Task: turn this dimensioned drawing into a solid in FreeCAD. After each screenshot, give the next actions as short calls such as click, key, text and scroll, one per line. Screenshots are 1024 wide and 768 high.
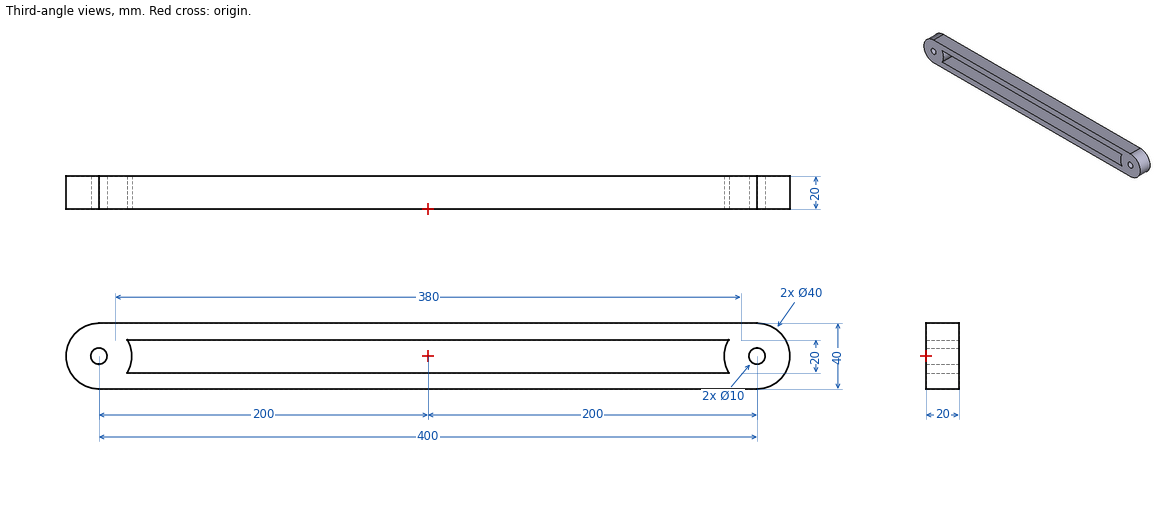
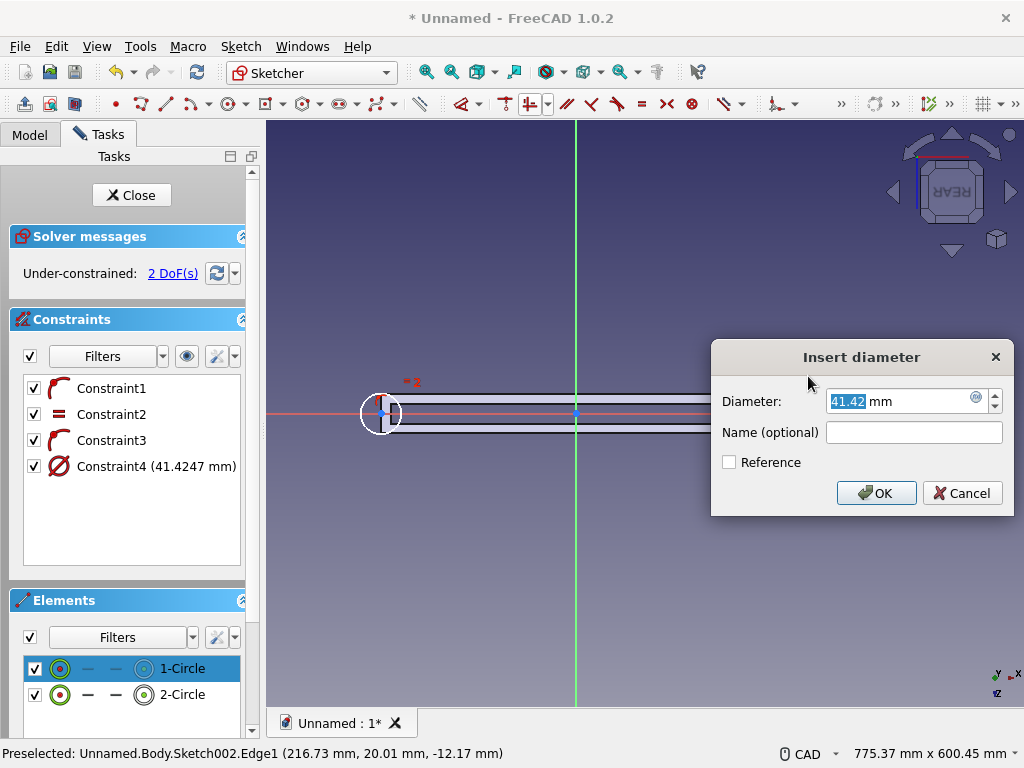
text(40)
key(Return)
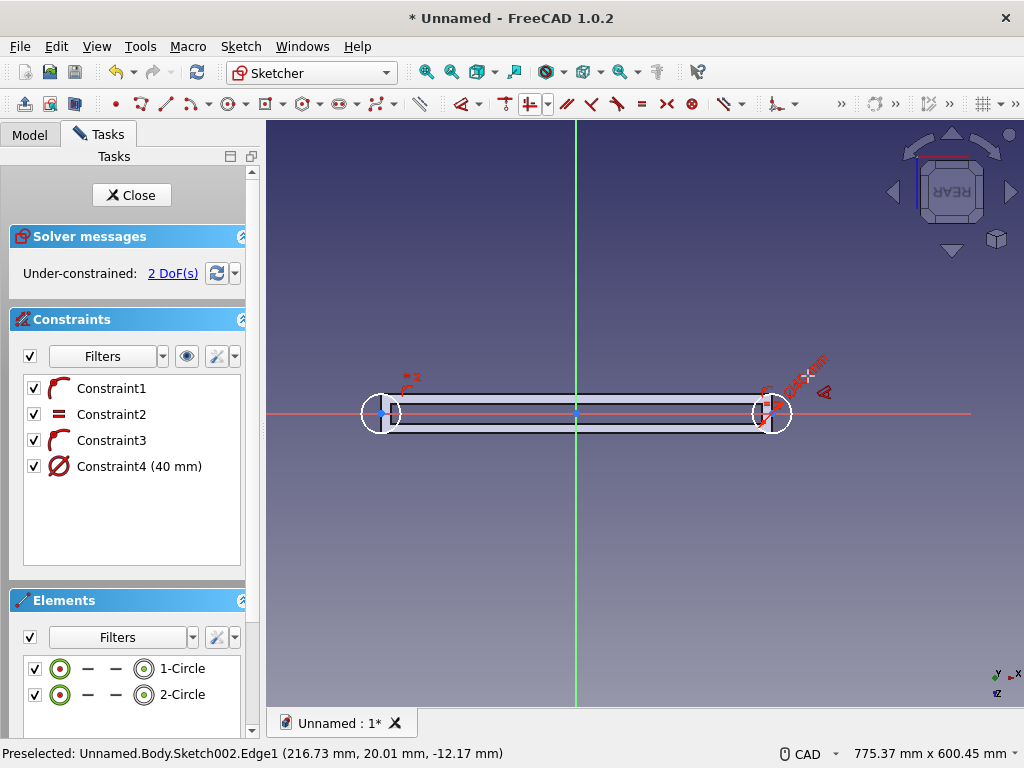
click(772, 414)
click(674, 448)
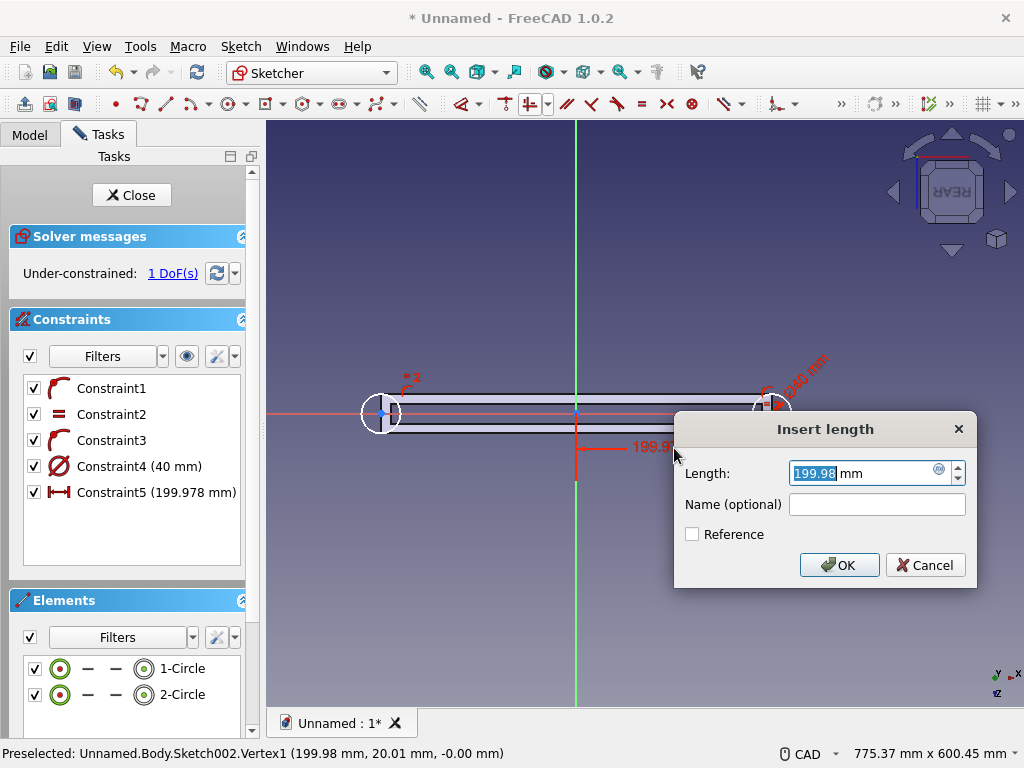
text(200)
key(Return)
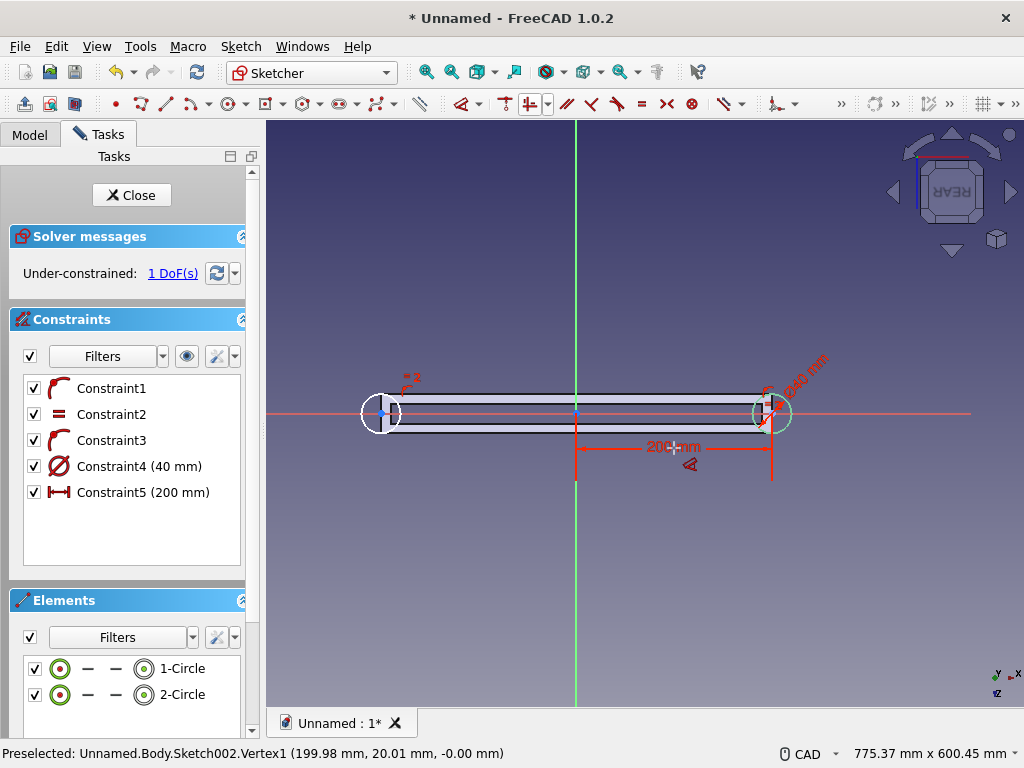
click(381, 414)
click(479, 448)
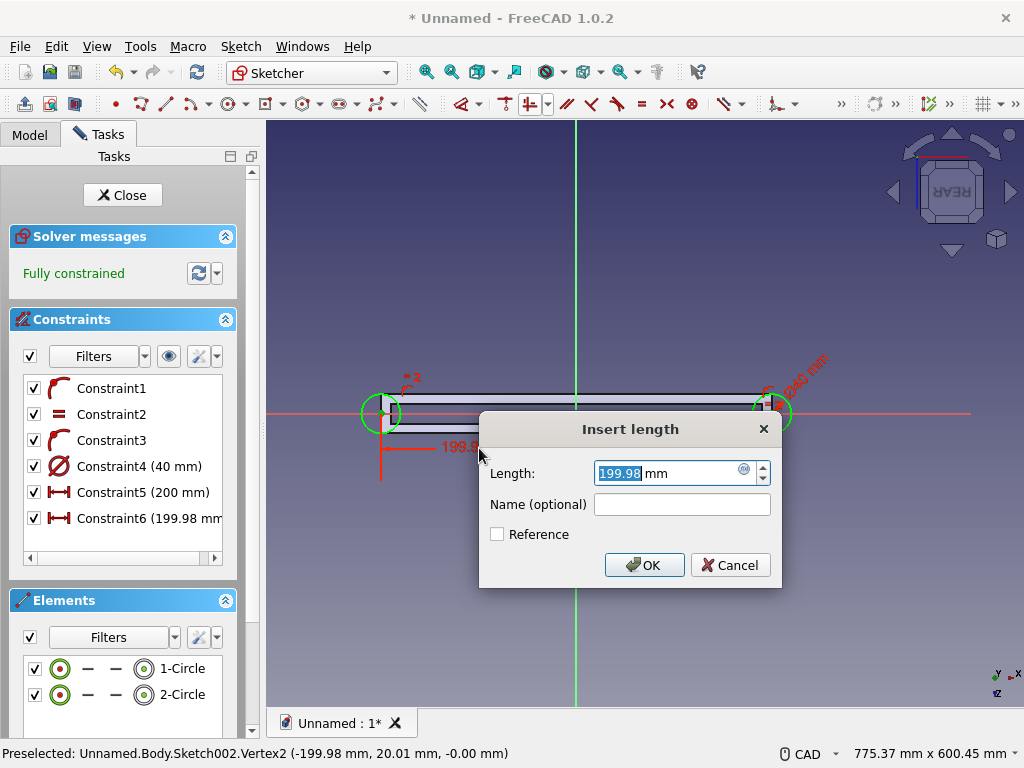
text(200)
key(Return)
key(Escape)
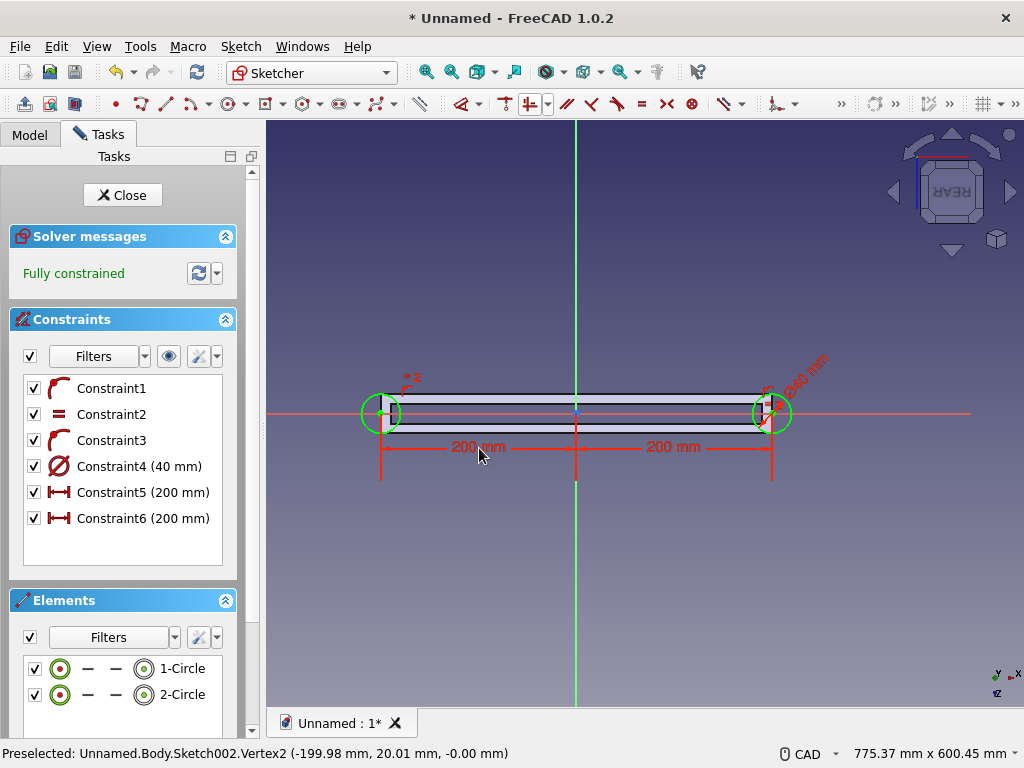
click(123, 195)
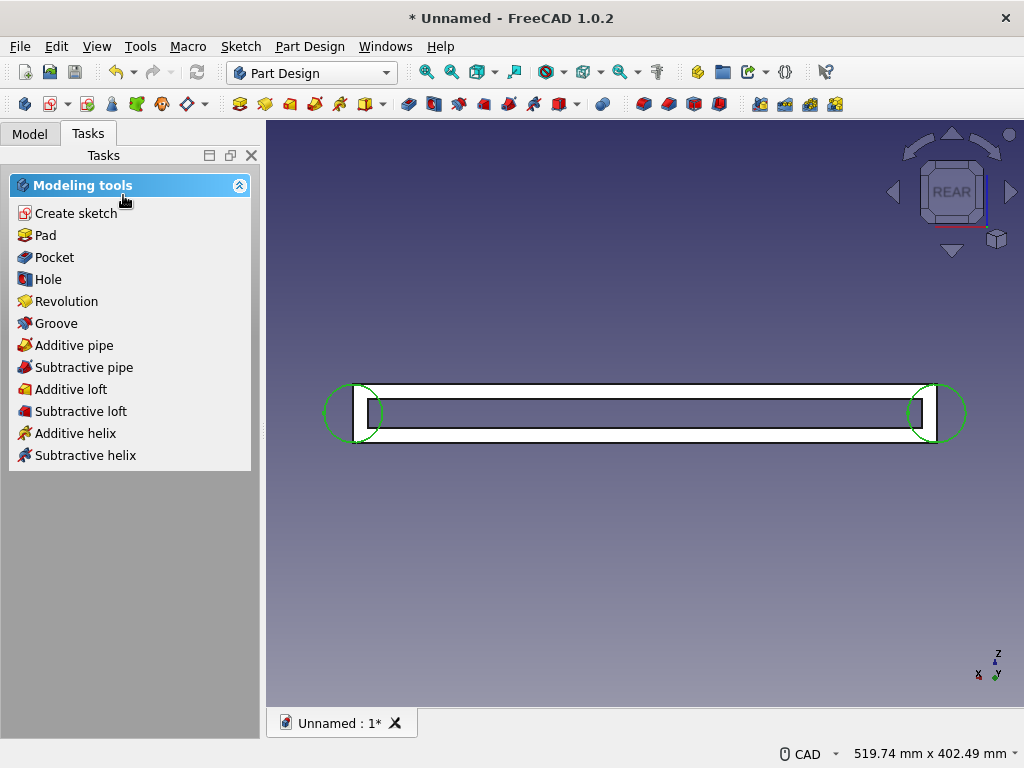
click(240, 104)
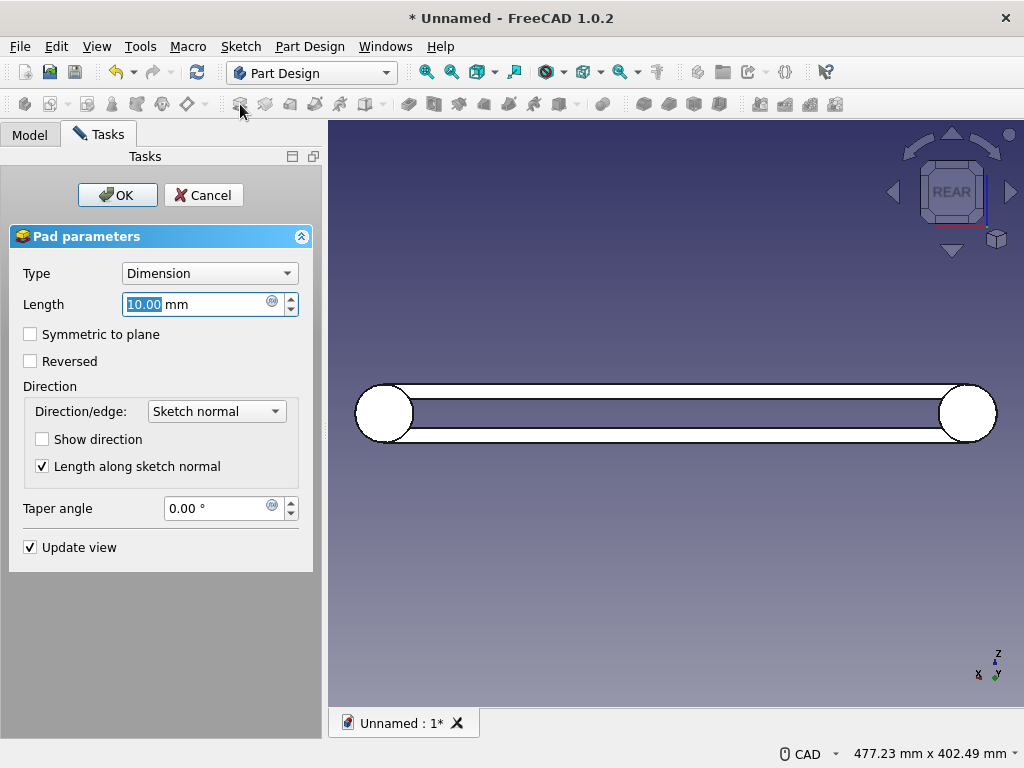
text(20)
key(Tab)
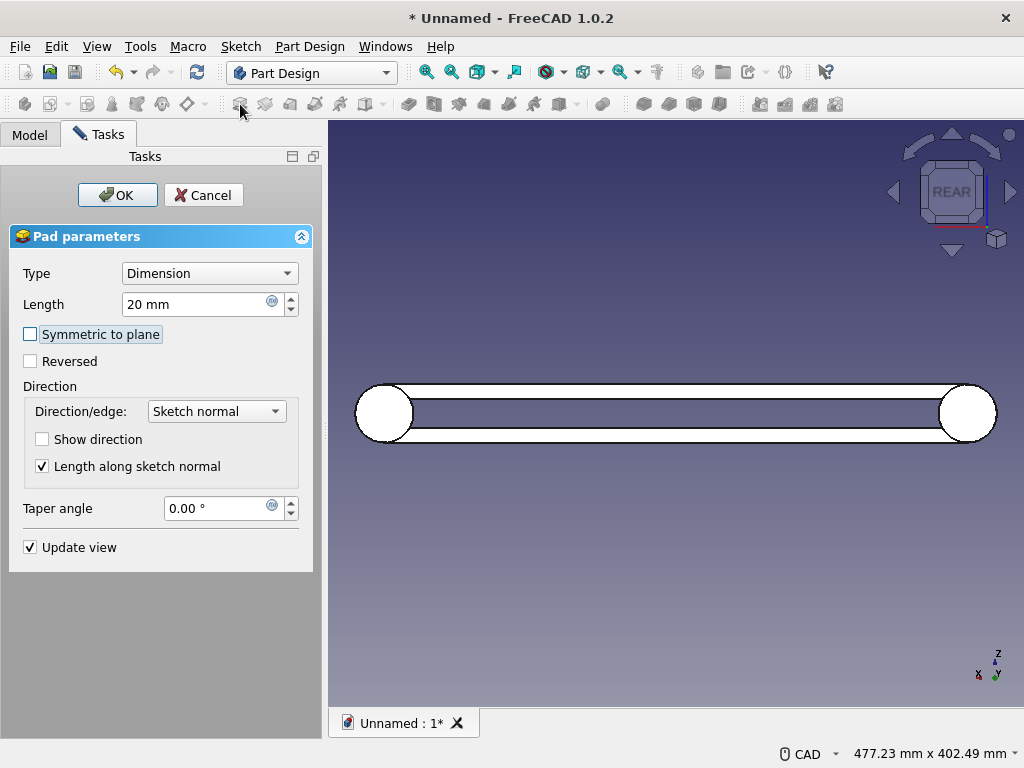
click(31, 361)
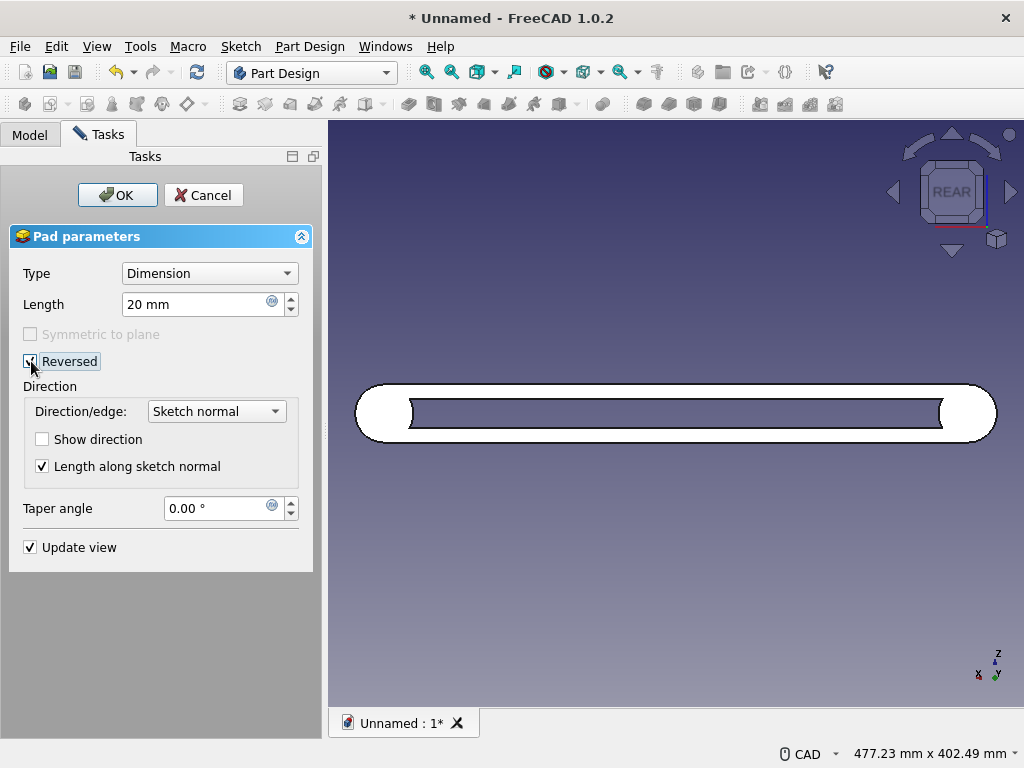
click(118, 195)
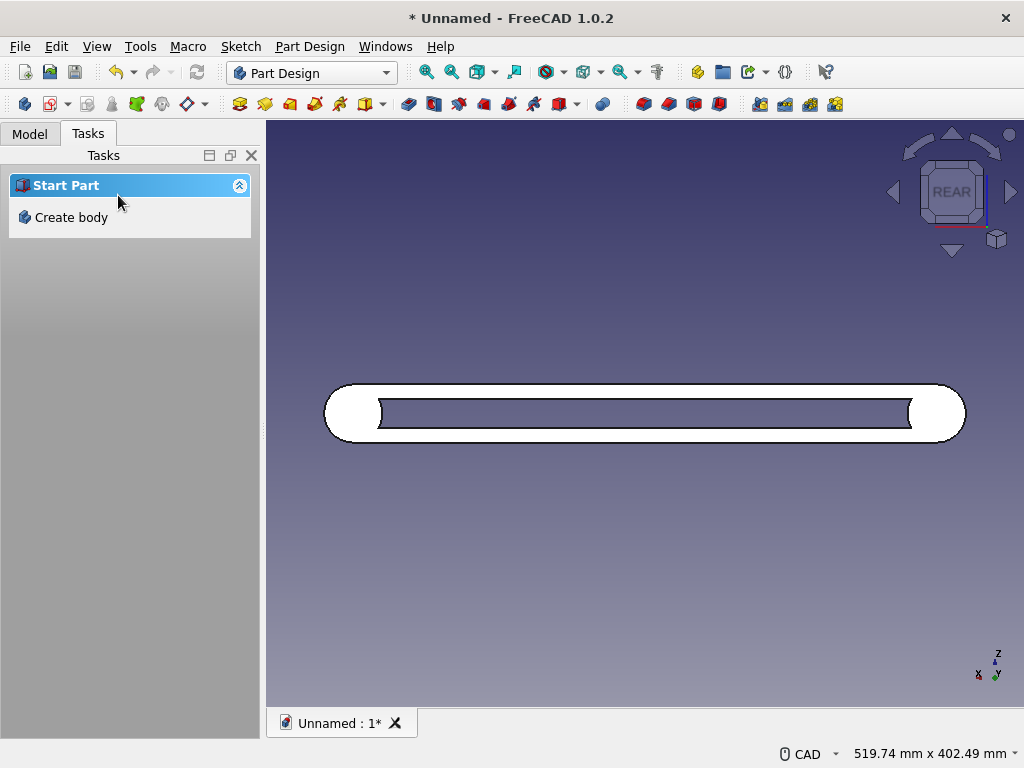
click(370, 412)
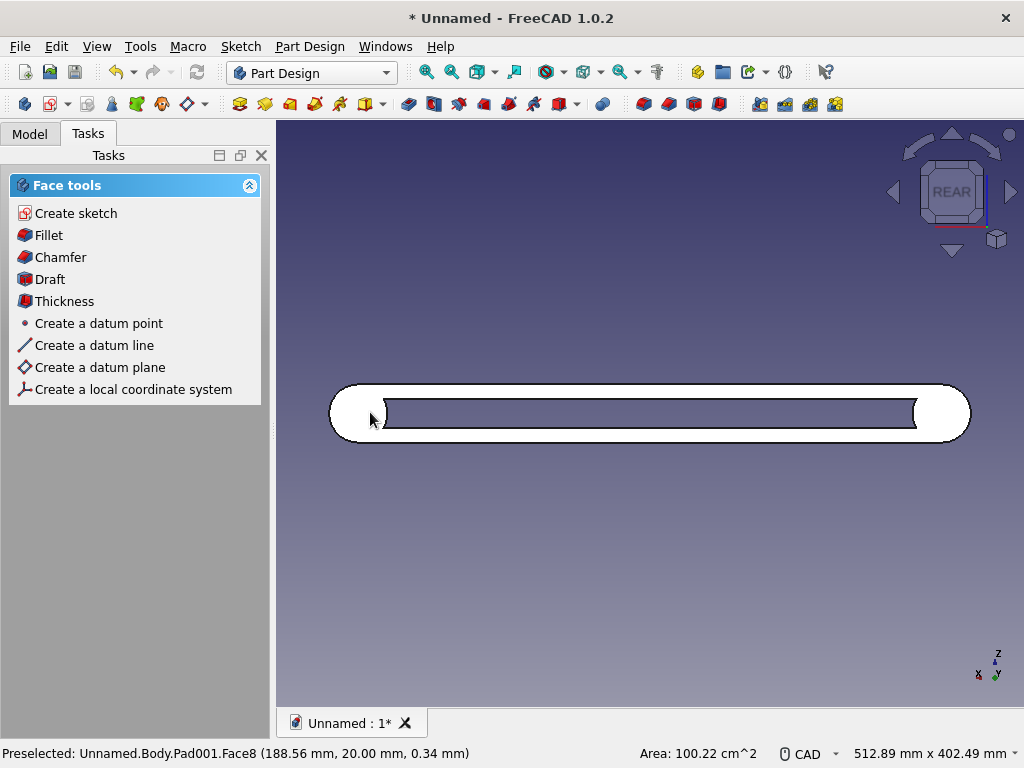
click(50, 104)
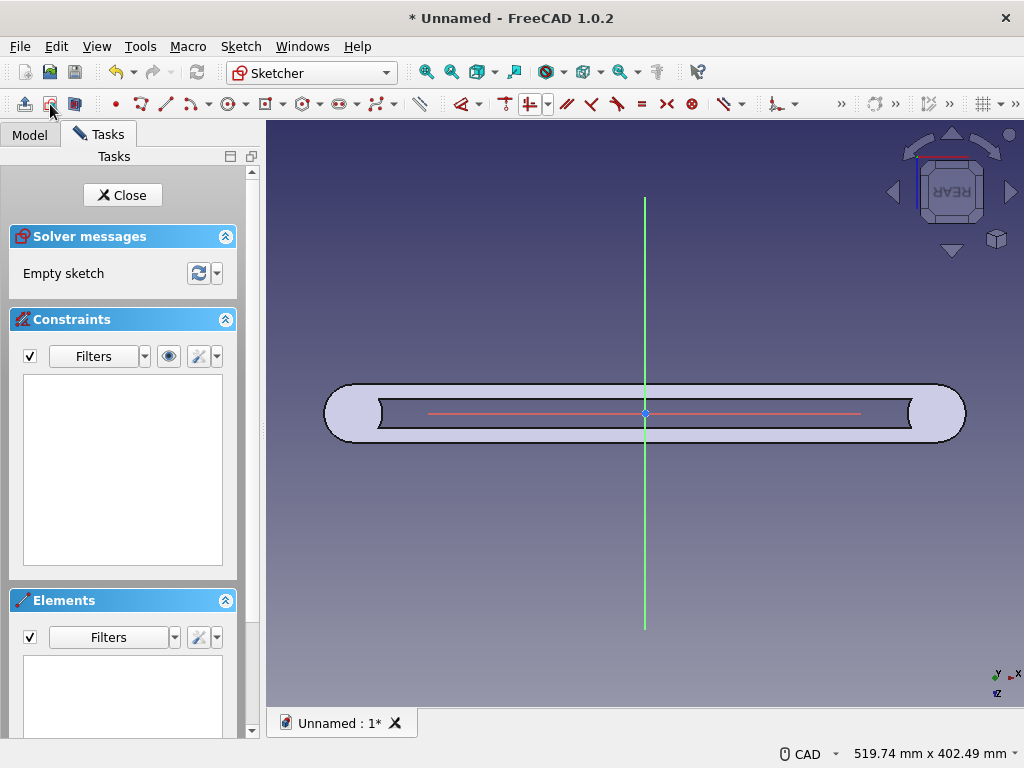
scroll(437, 414, down, 2)